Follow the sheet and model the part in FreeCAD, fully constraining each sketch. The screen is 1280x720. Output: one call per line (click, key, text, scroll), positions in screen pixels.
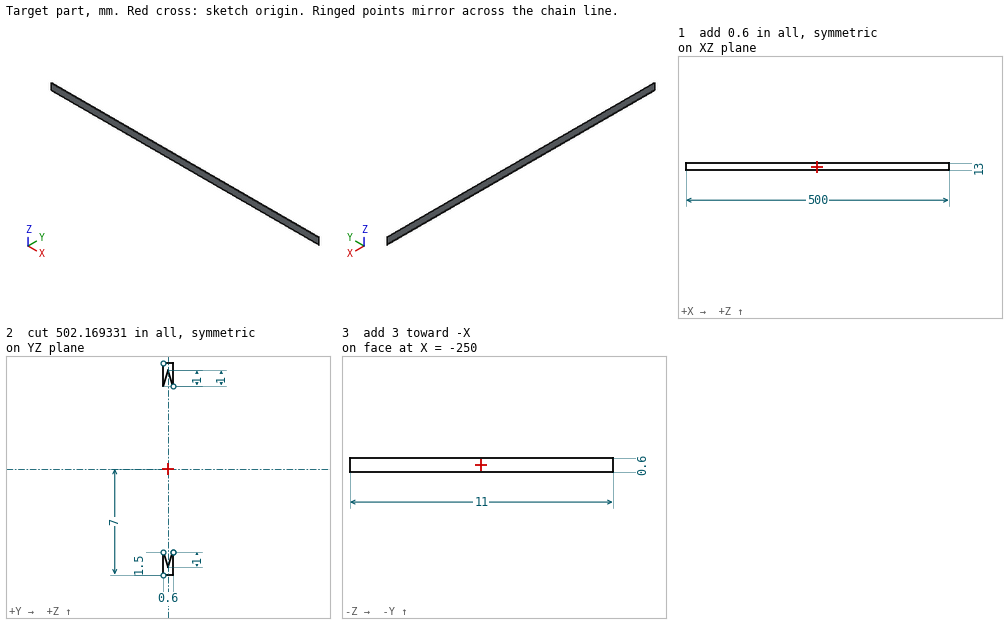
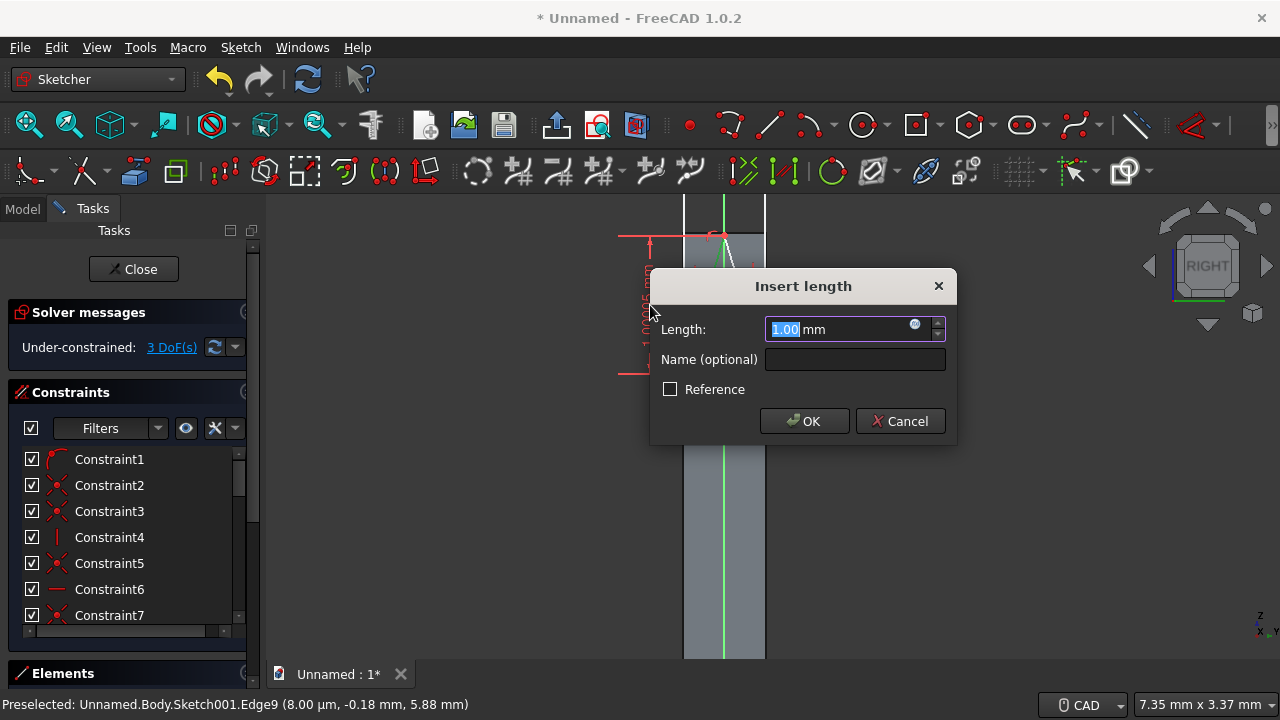
text(1)
key(Return)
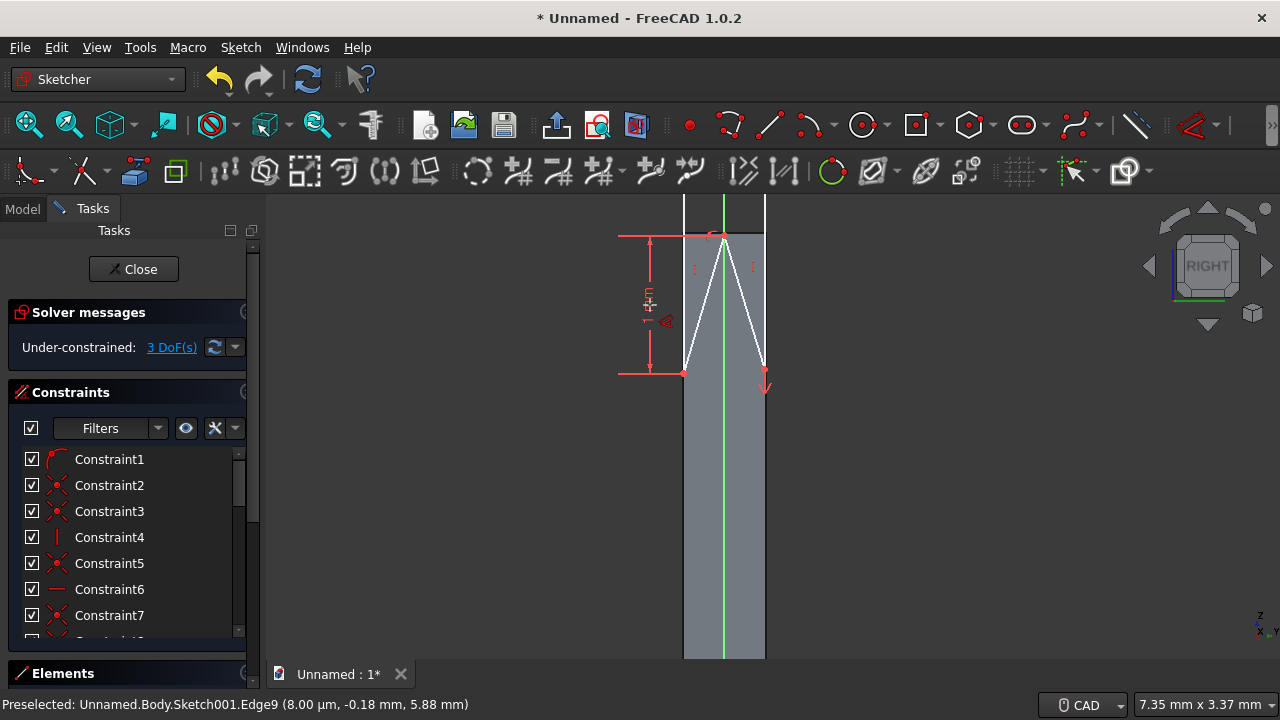
click(736, 276)
click(799, 302)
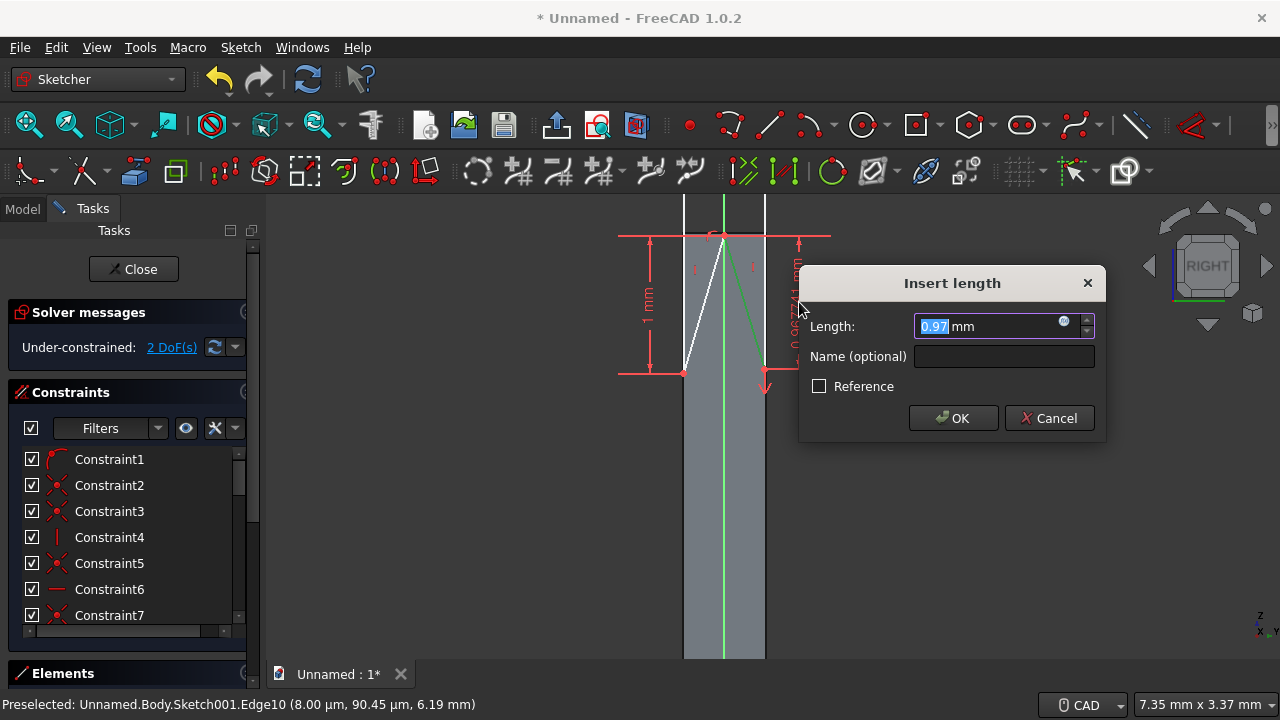
text(1)
key(Return)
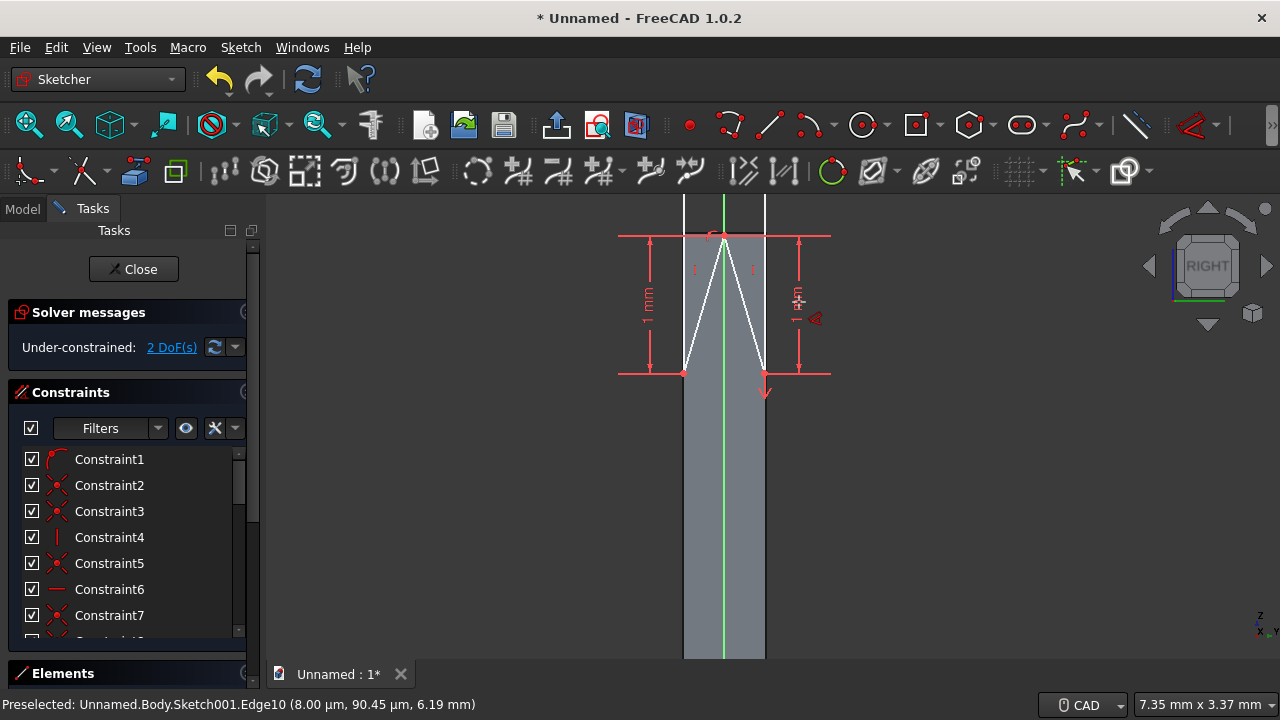
scroll(701, 316, down, 10)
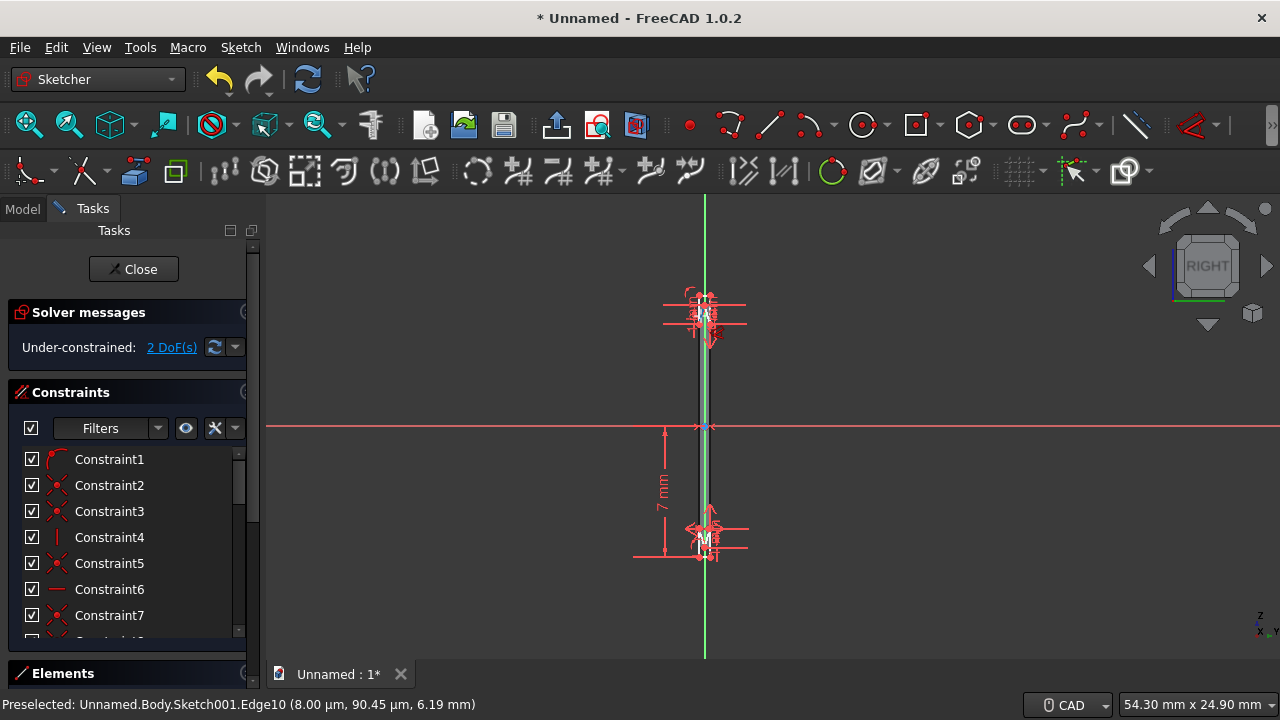
scroll(699, 537, up, 9)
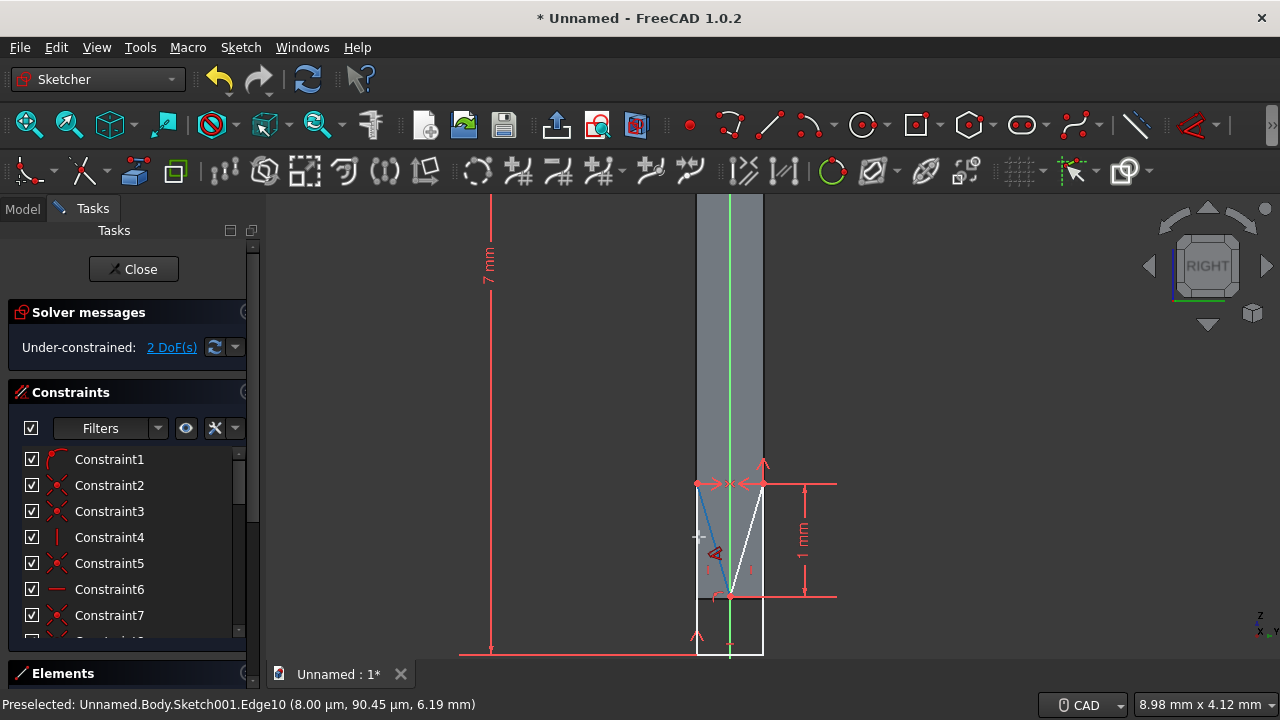
click(697, 535)
click(663, 557)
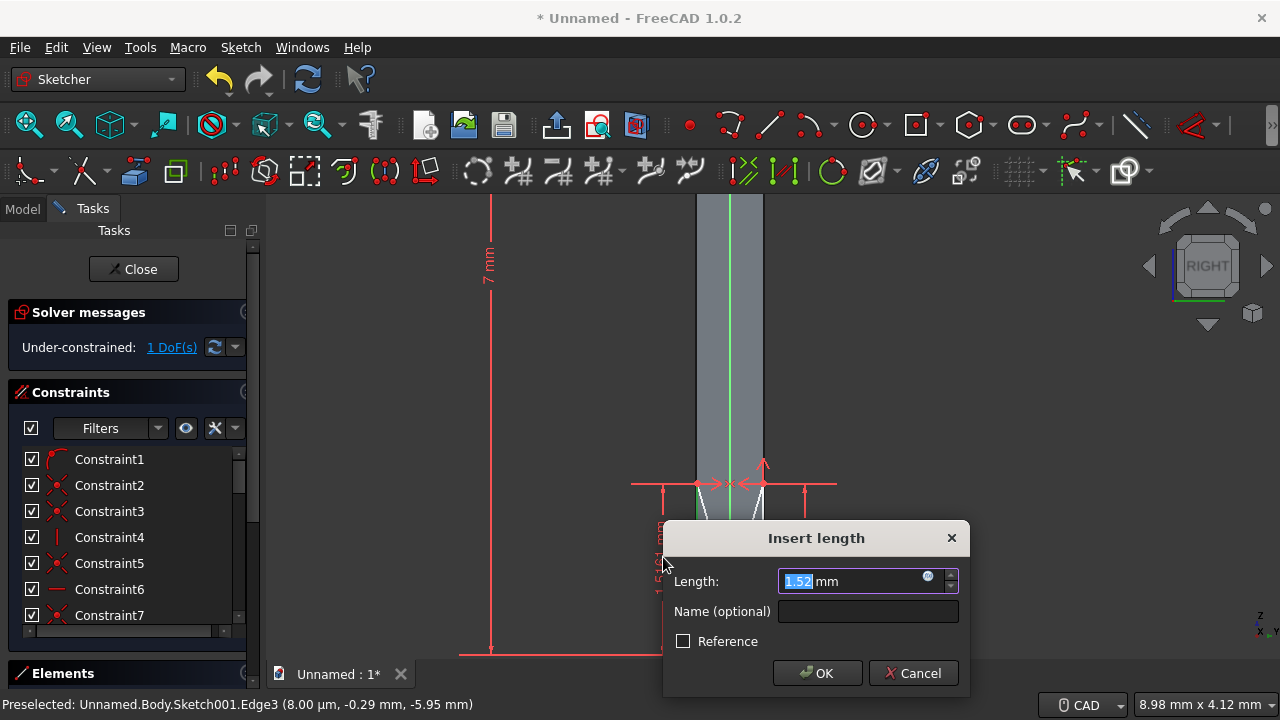
text(1.5)
key(Return)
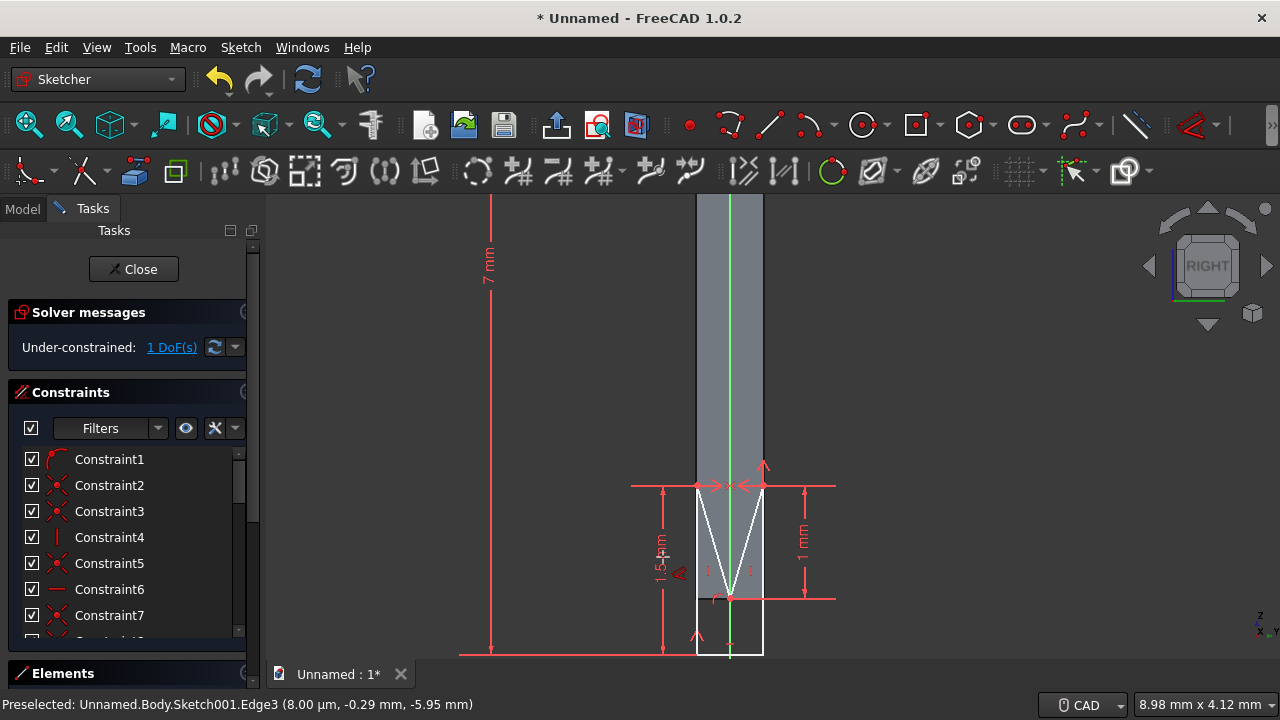
scroll(699, 538, down, 9)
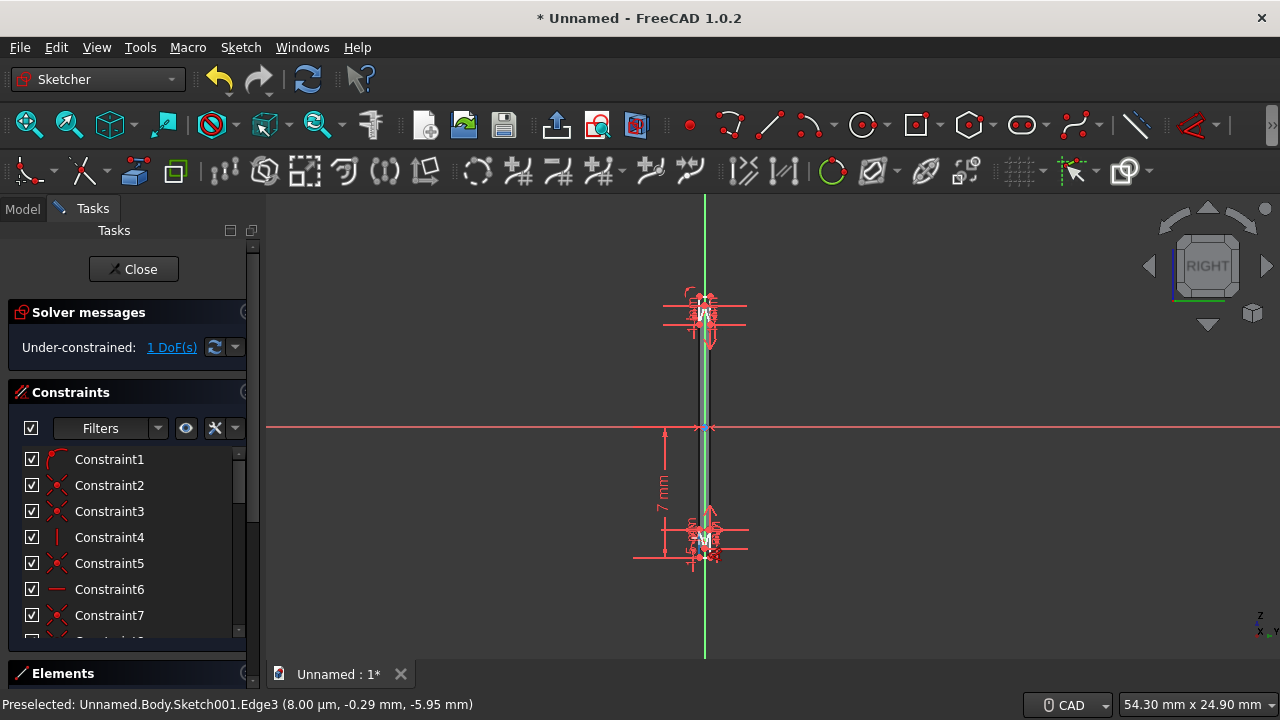
scroll(702, 558, up, 10)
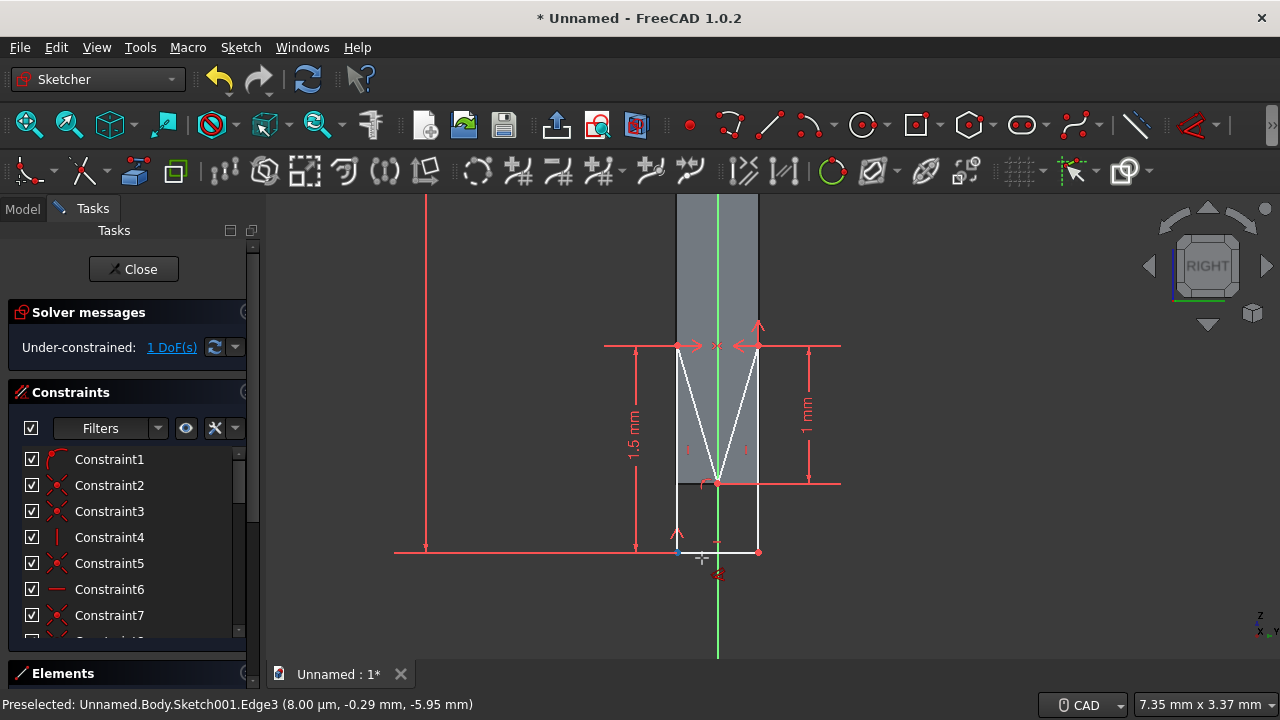
click(702, 553)
click(699, 587)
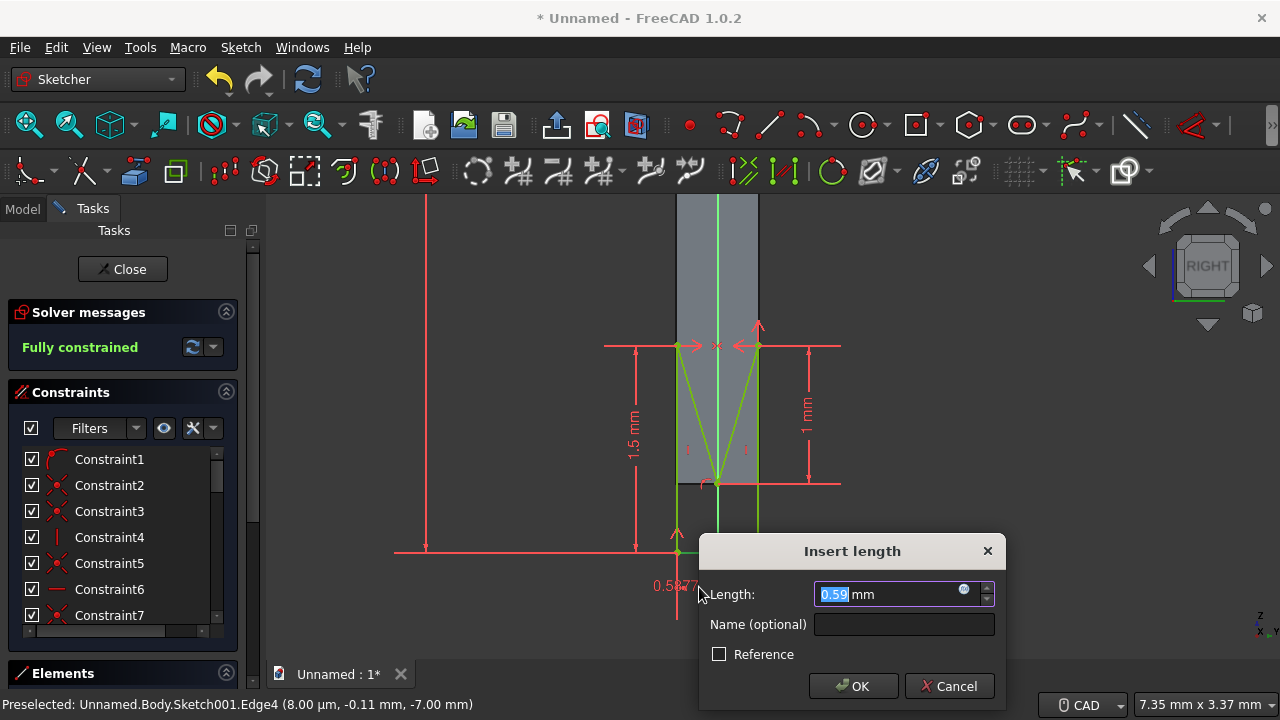
text(0.6)
key(Return)
key(Escape)